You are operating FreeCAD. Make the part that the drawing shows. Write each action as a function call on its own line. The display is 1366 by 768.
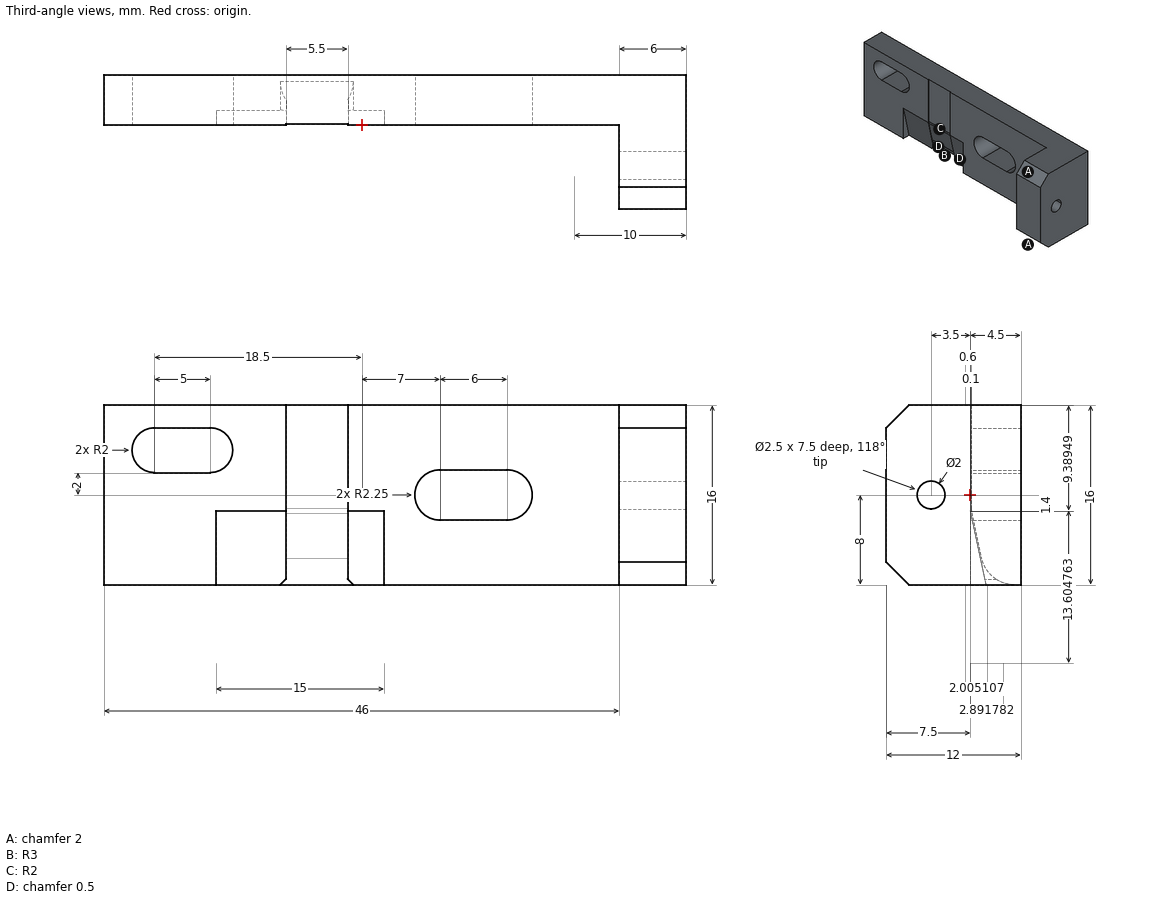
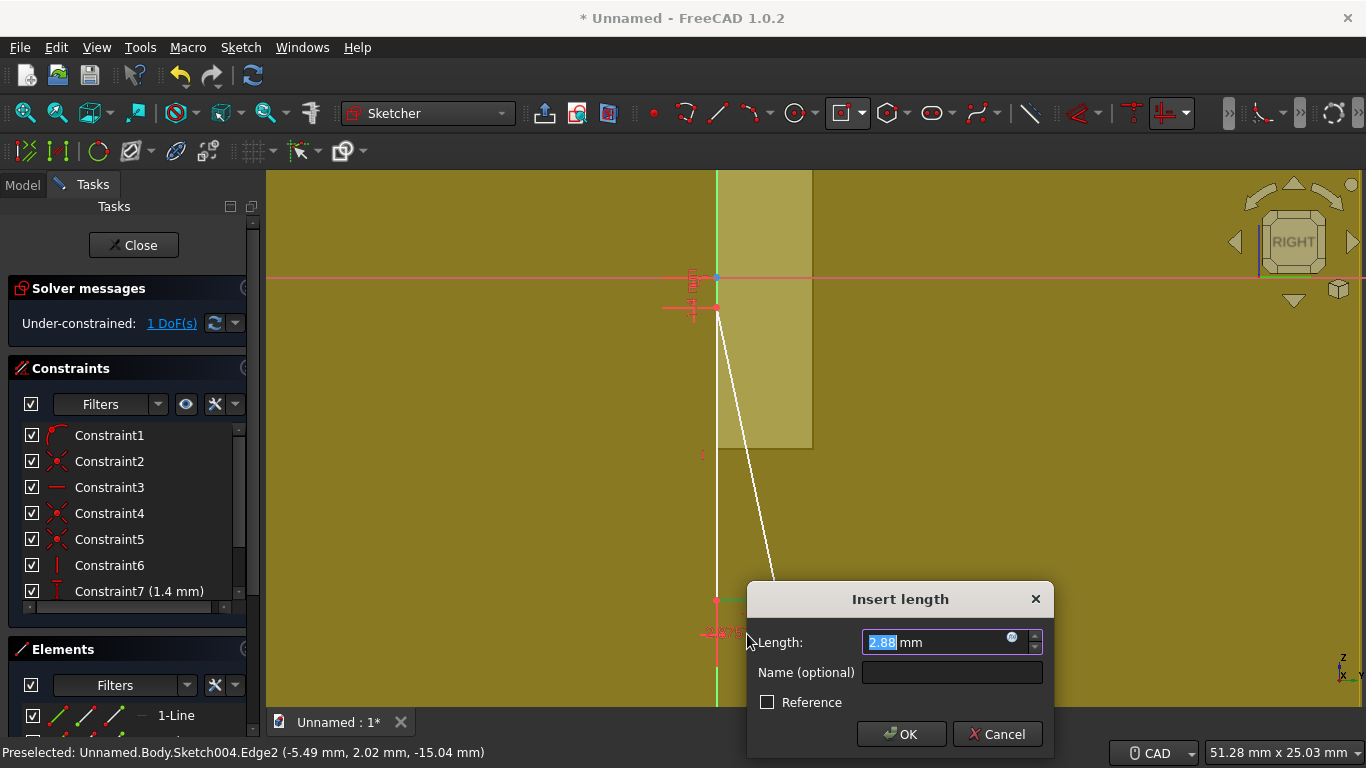
text(2.891782)
key(Return)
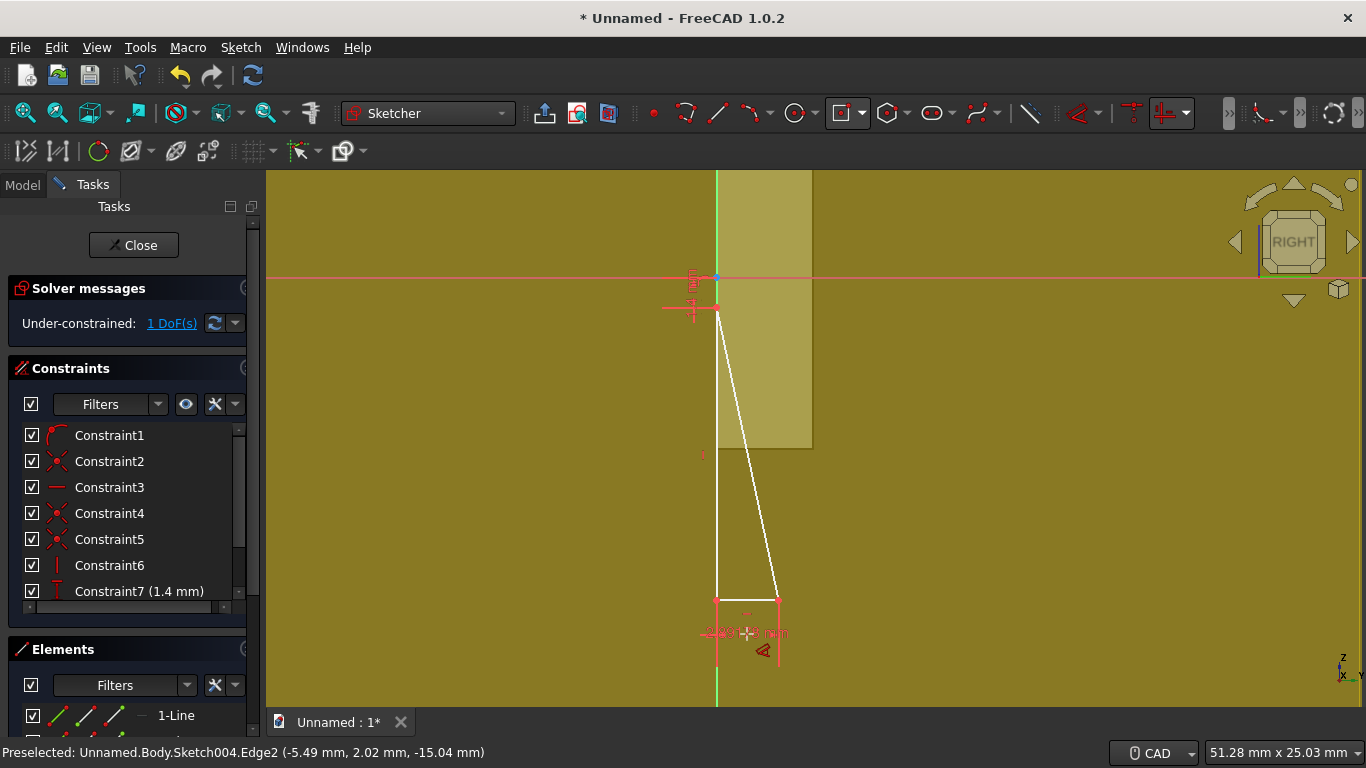
click(717, 513)
click(683, 454)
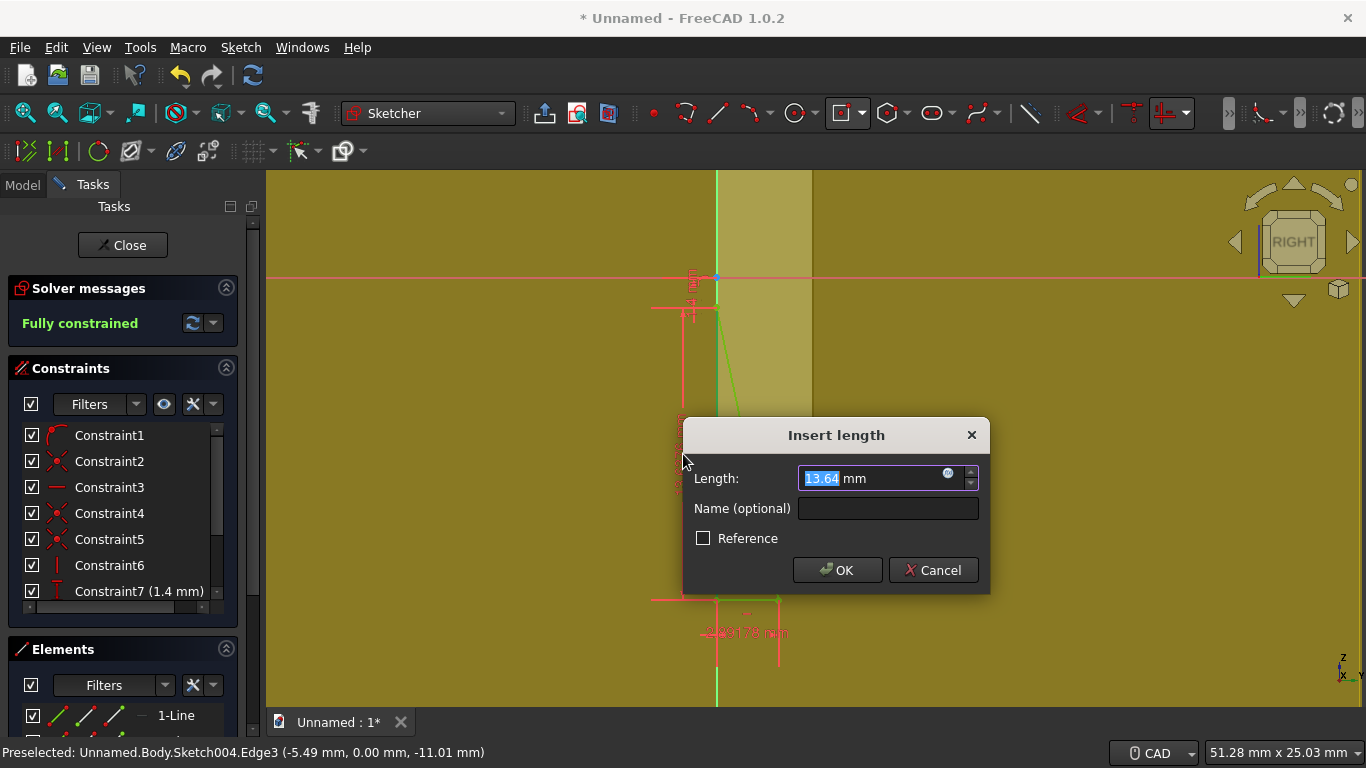
text(13.604763)
key(Return)
key(Escape)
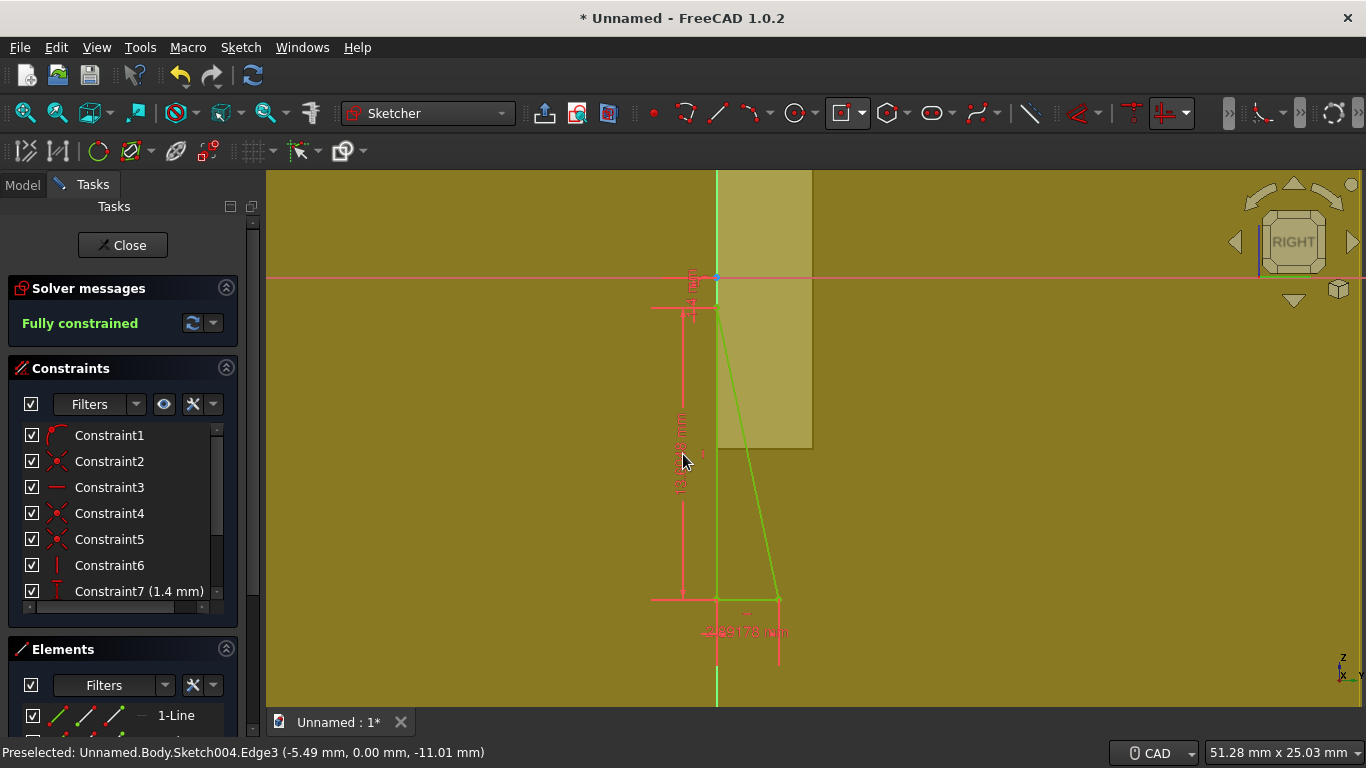
click(123, 245)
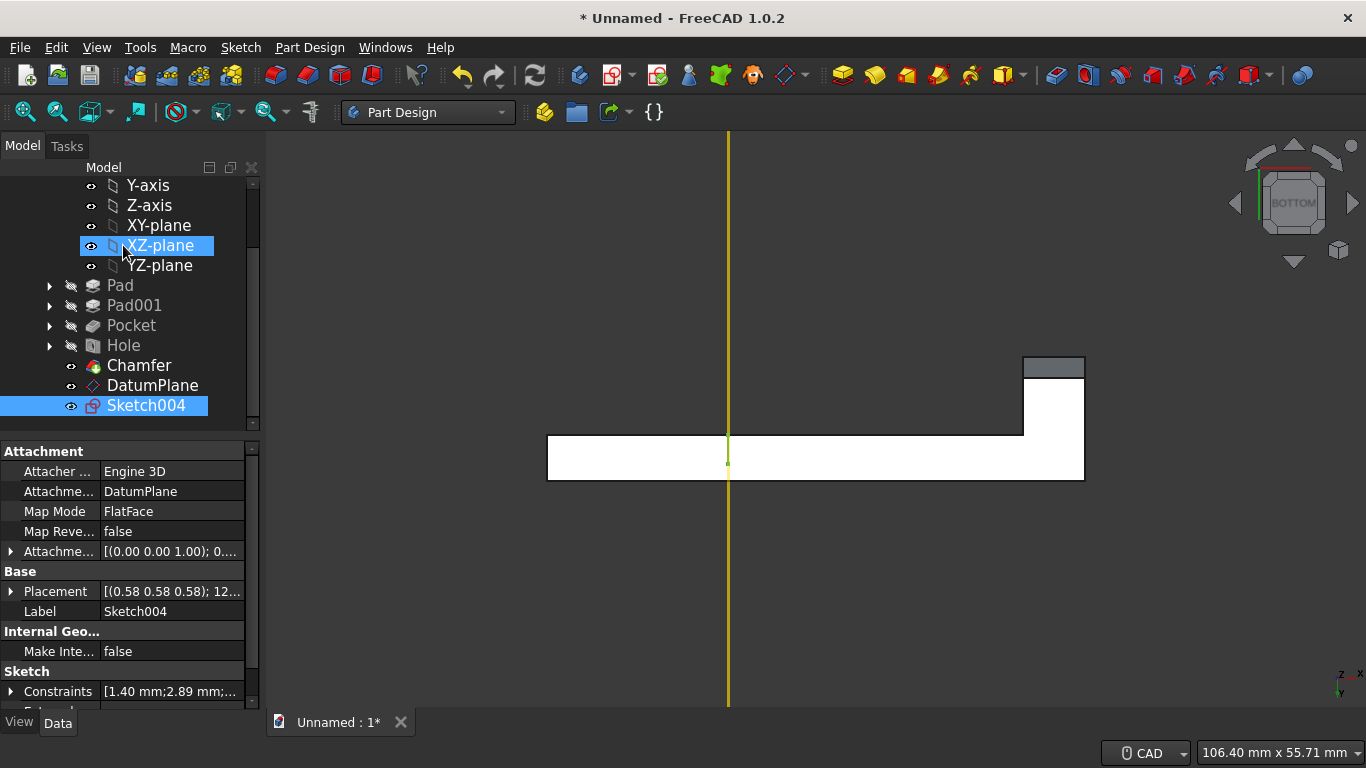
click(1058, 76)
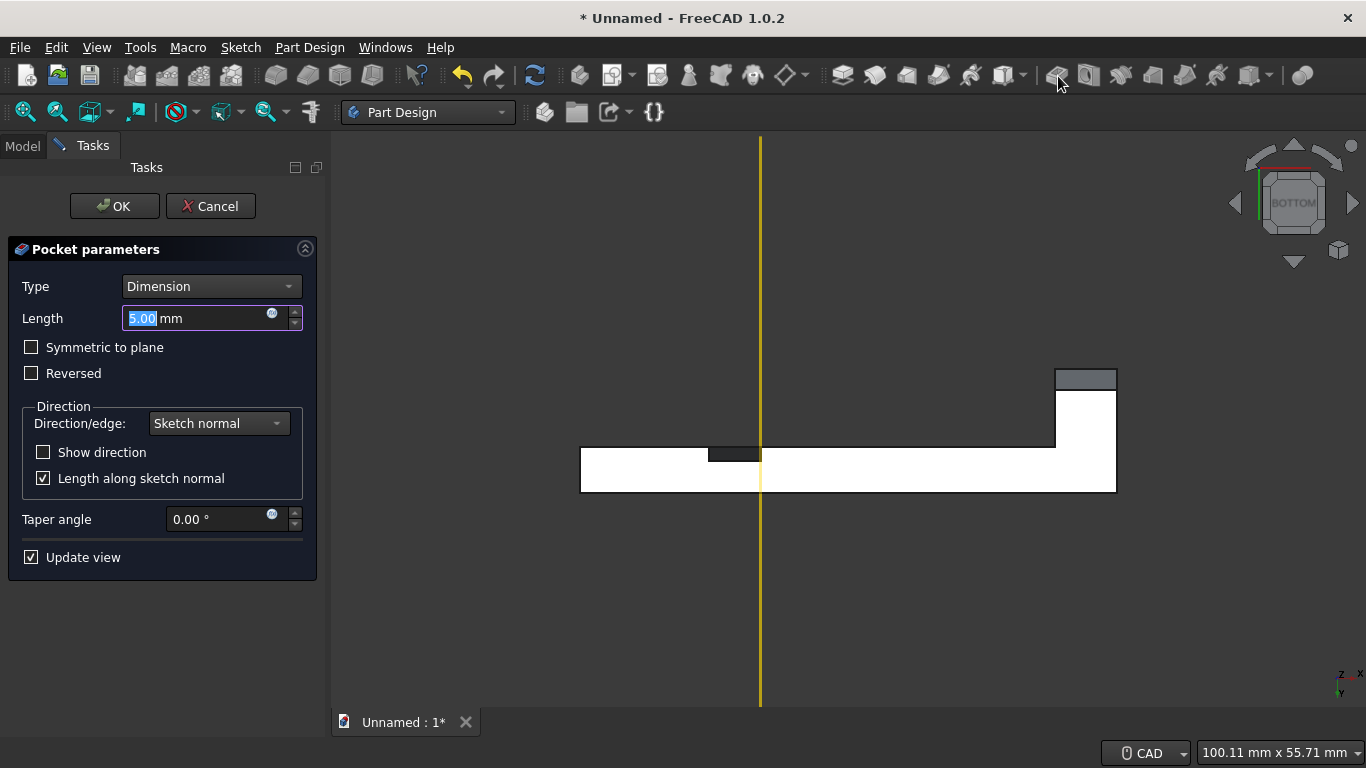
text(15)
key(Tab)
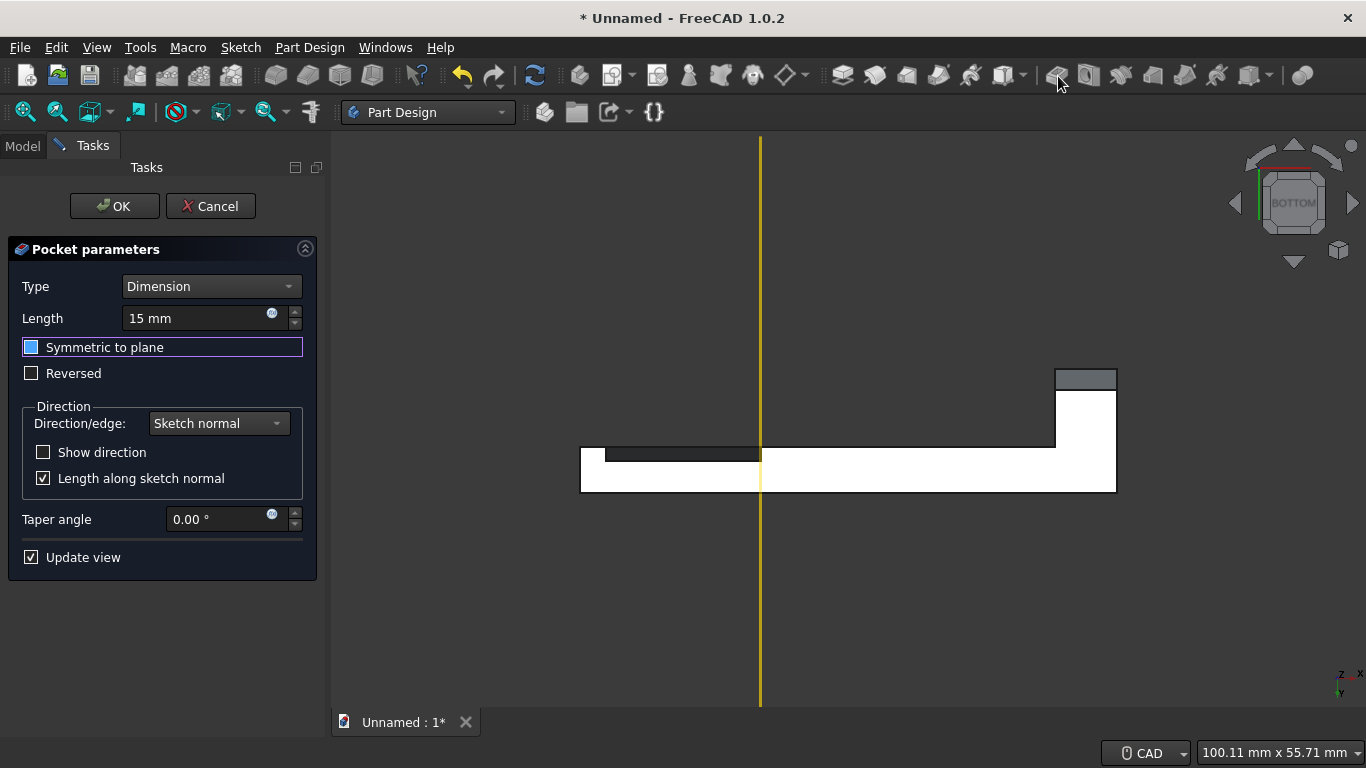
click(30, 347)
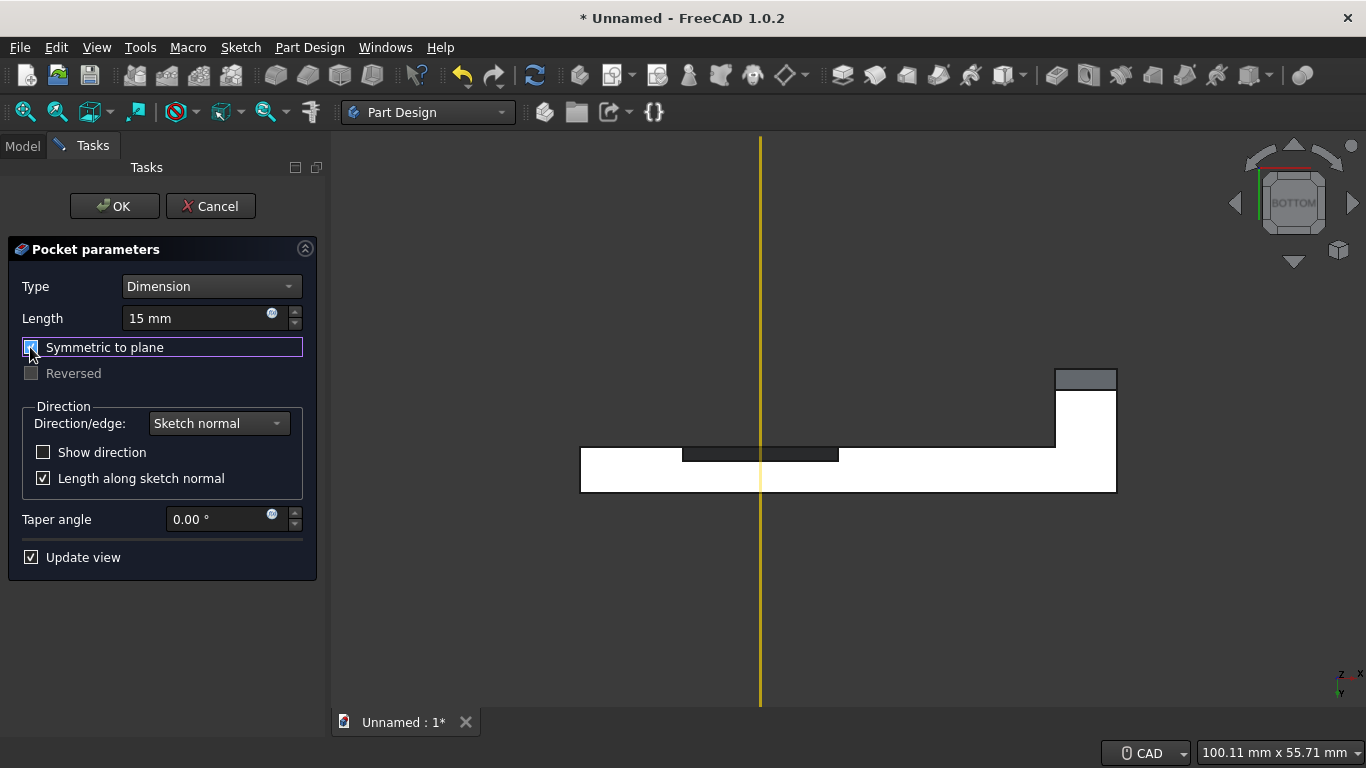
click(115, 206)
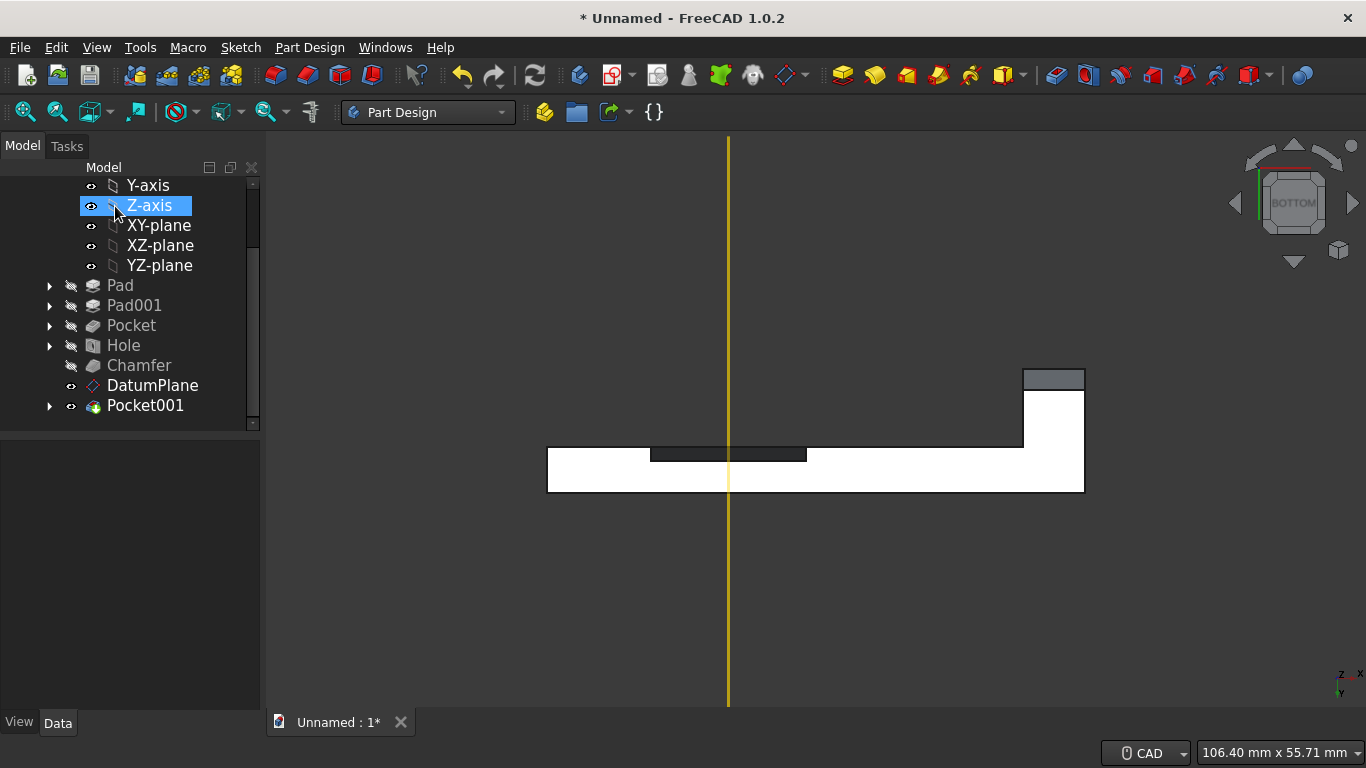
click(116, 386)
key(space)